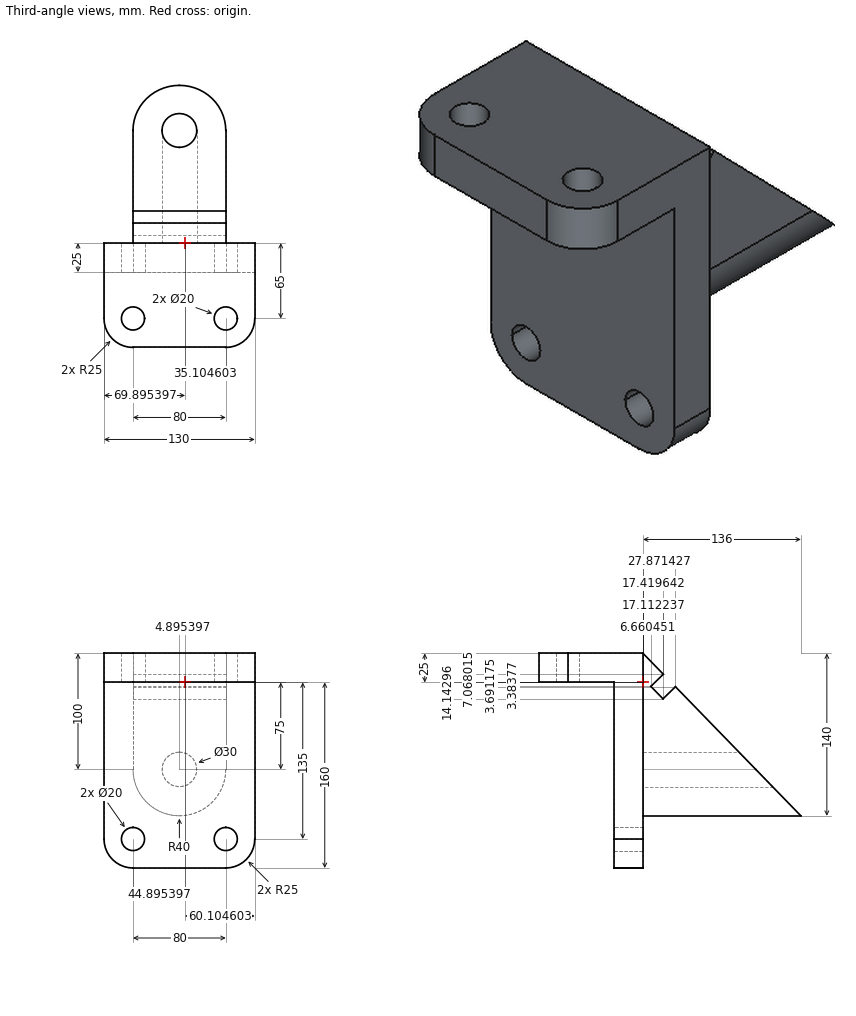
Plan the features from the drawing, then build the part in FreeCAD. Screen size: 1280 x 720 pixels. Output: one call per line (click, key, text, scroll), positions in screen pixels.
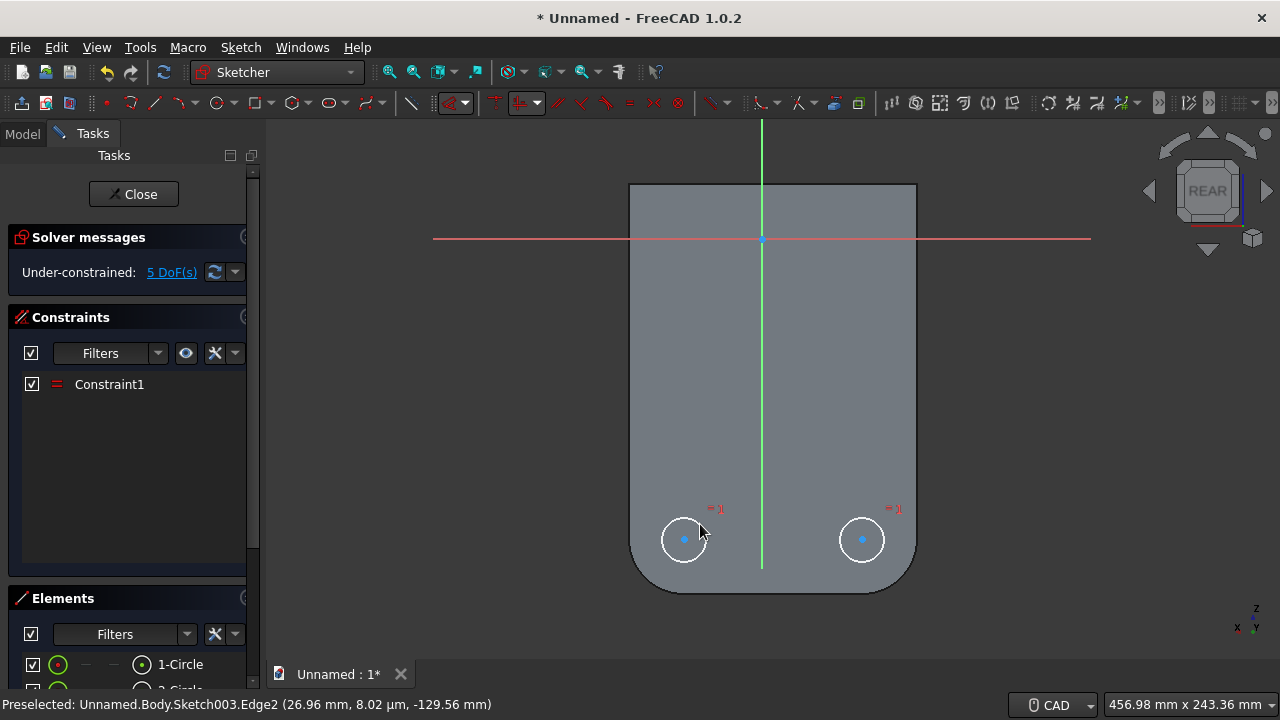
click(862, 540)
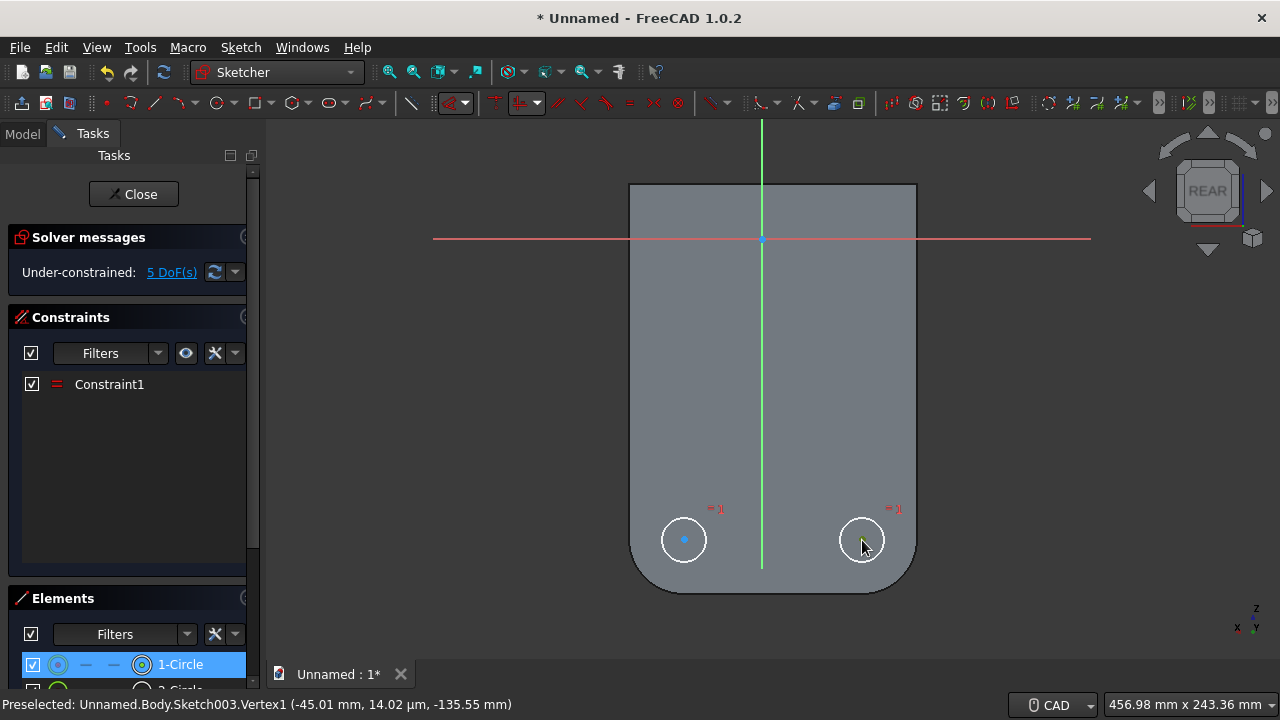
click(684, 540)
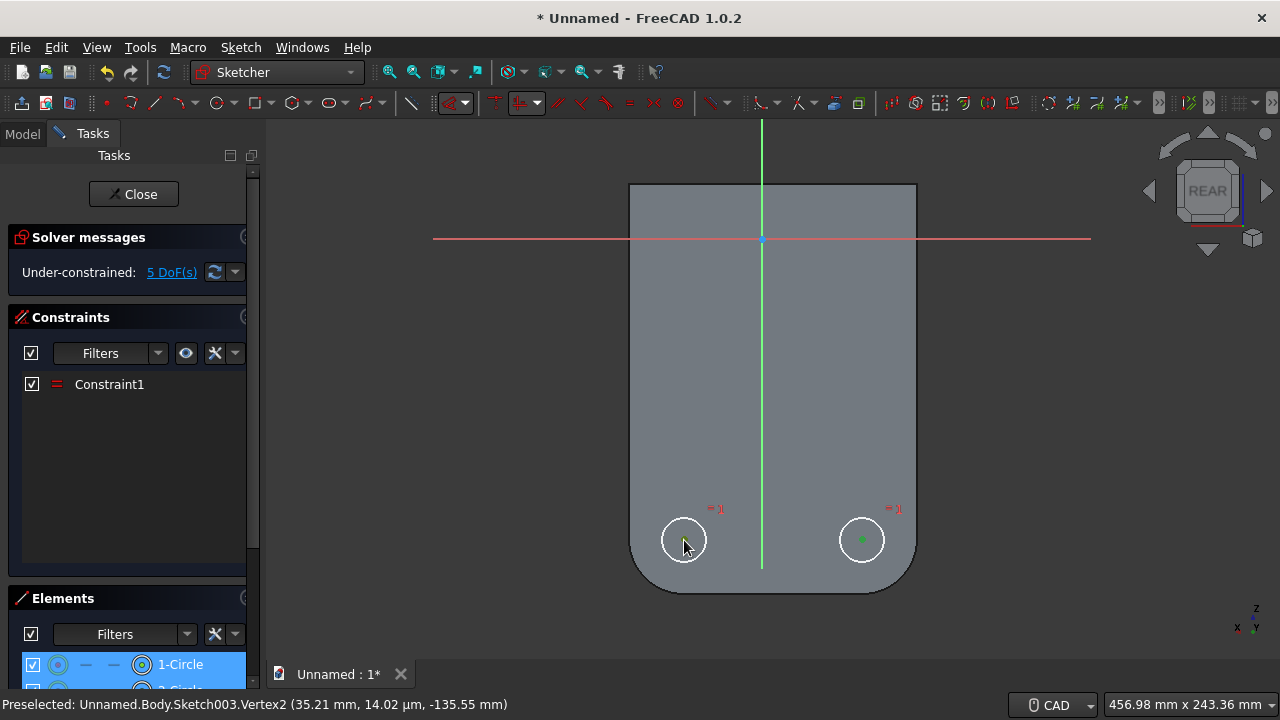
key(h)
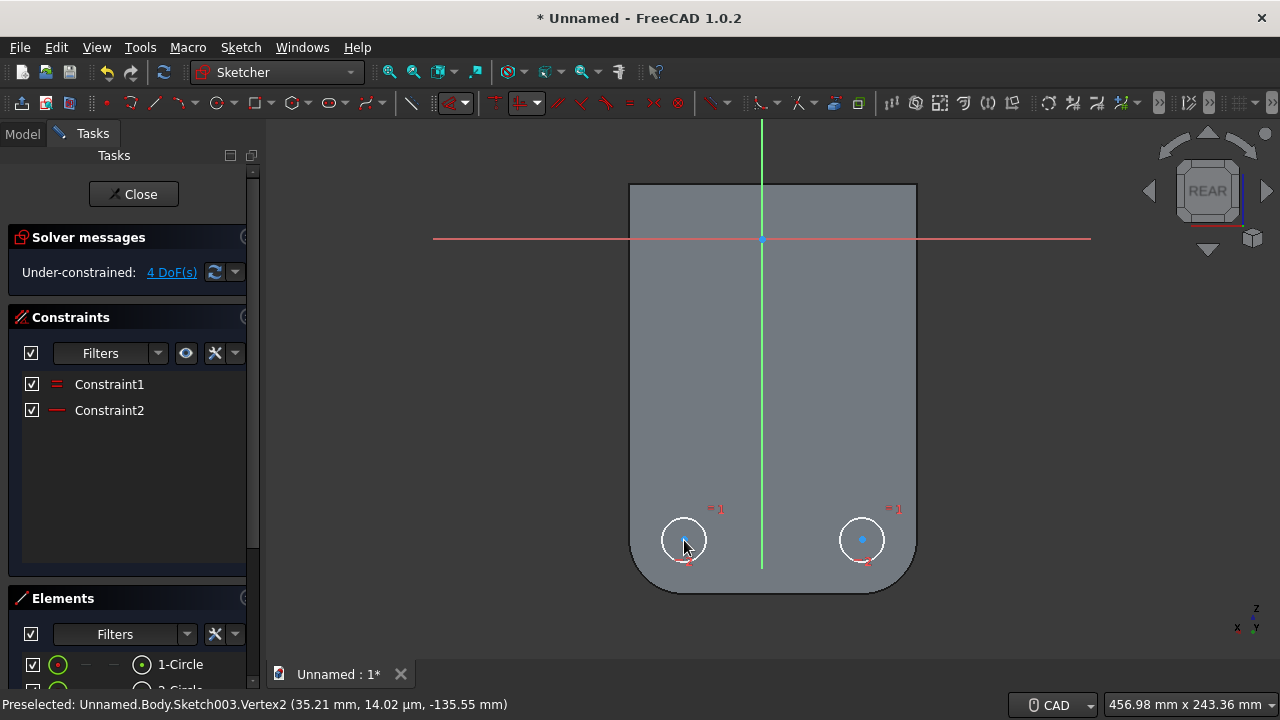
click(877, 524)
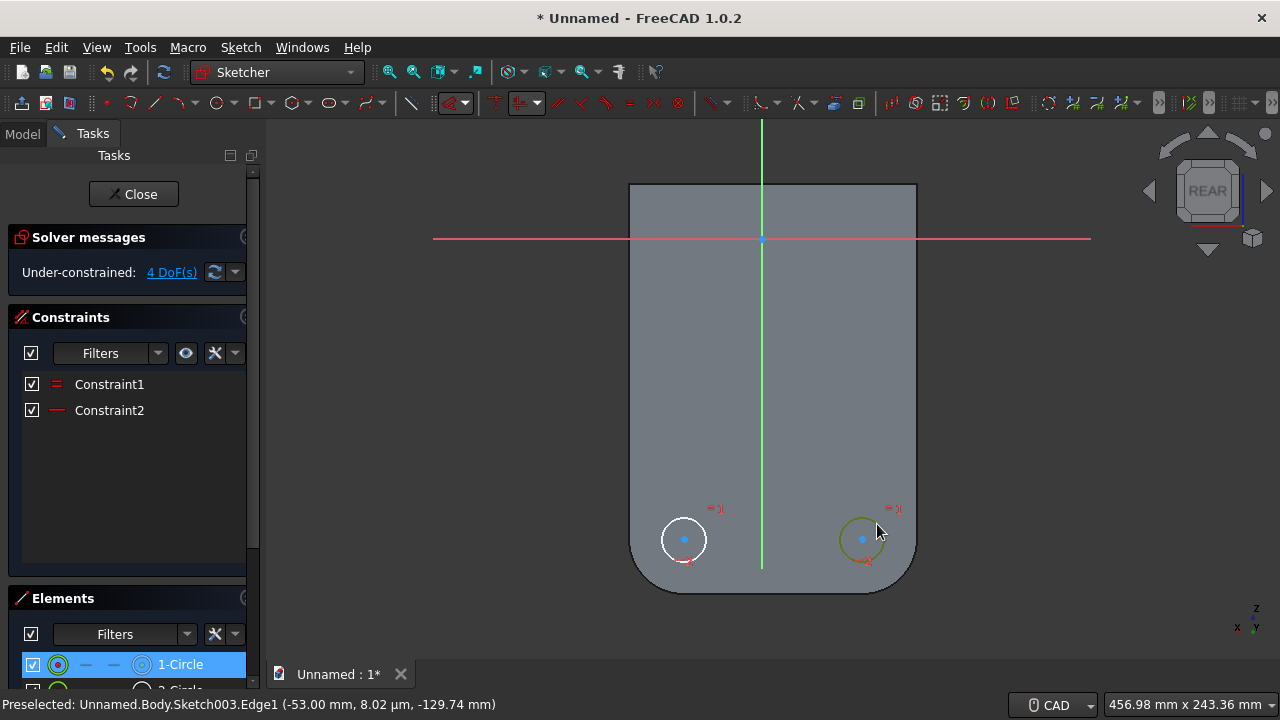
key(k)
key(o)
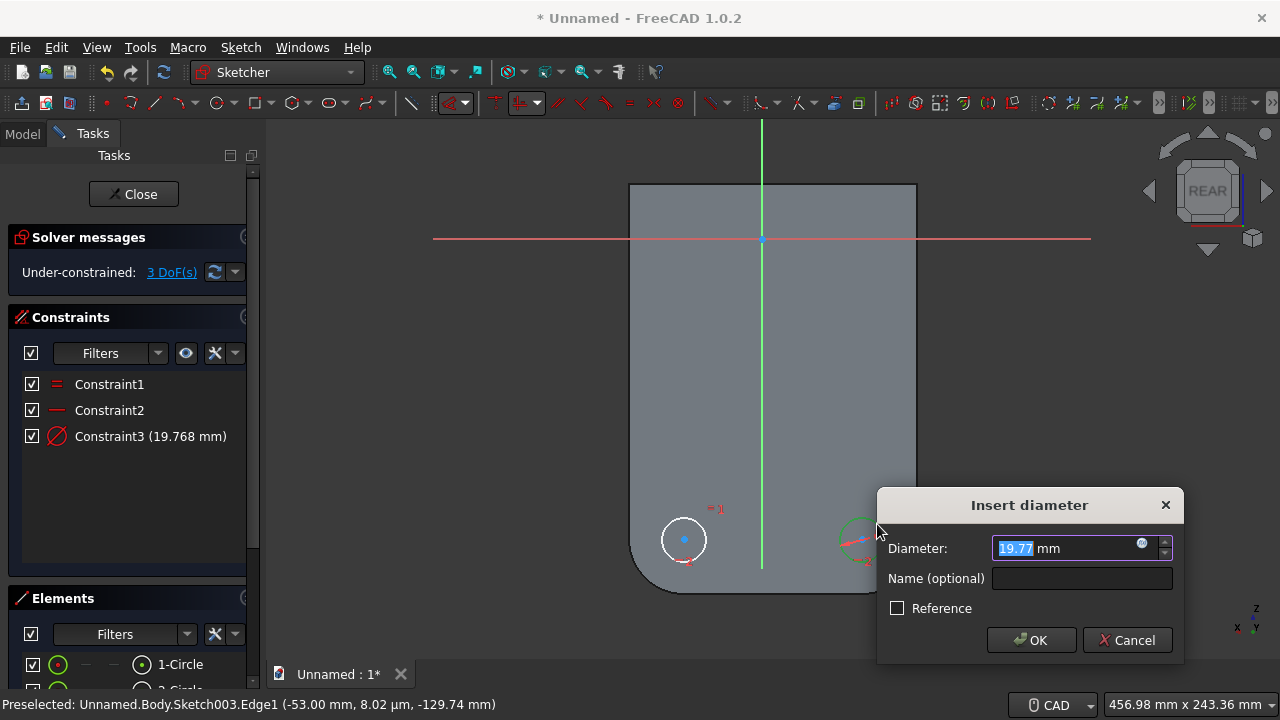
text(20)
key(Return)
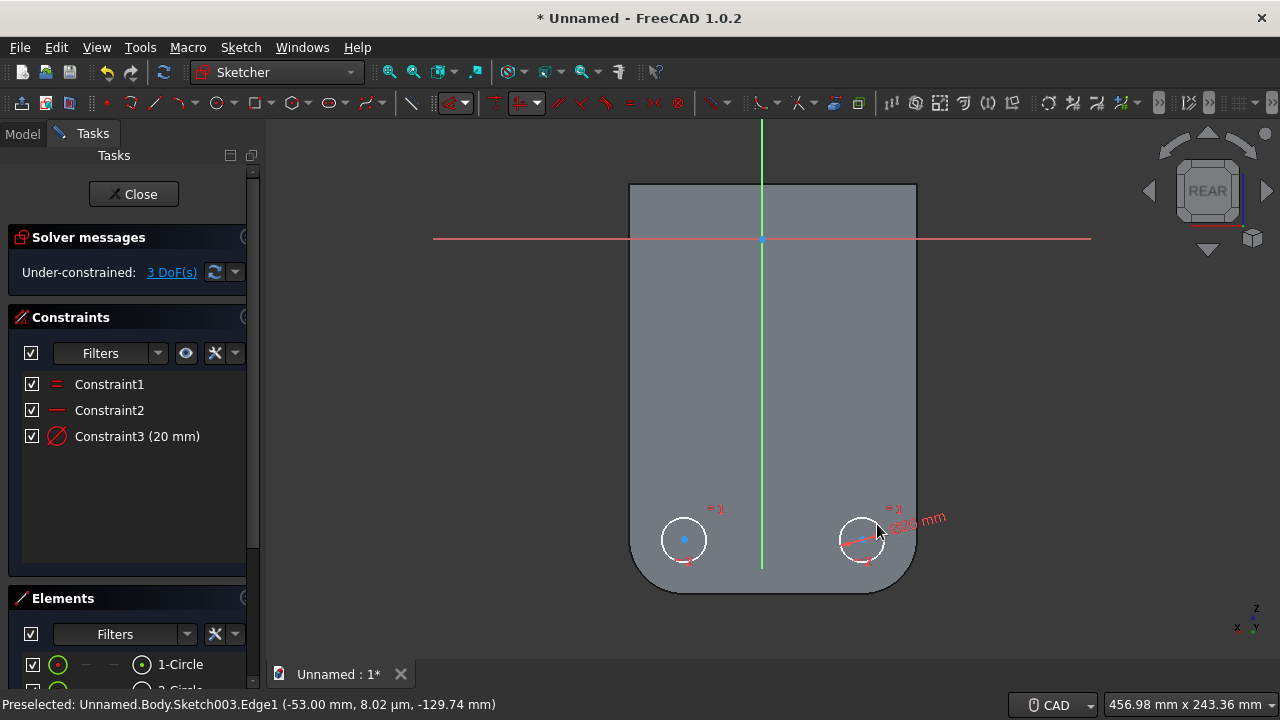
click(862, 540)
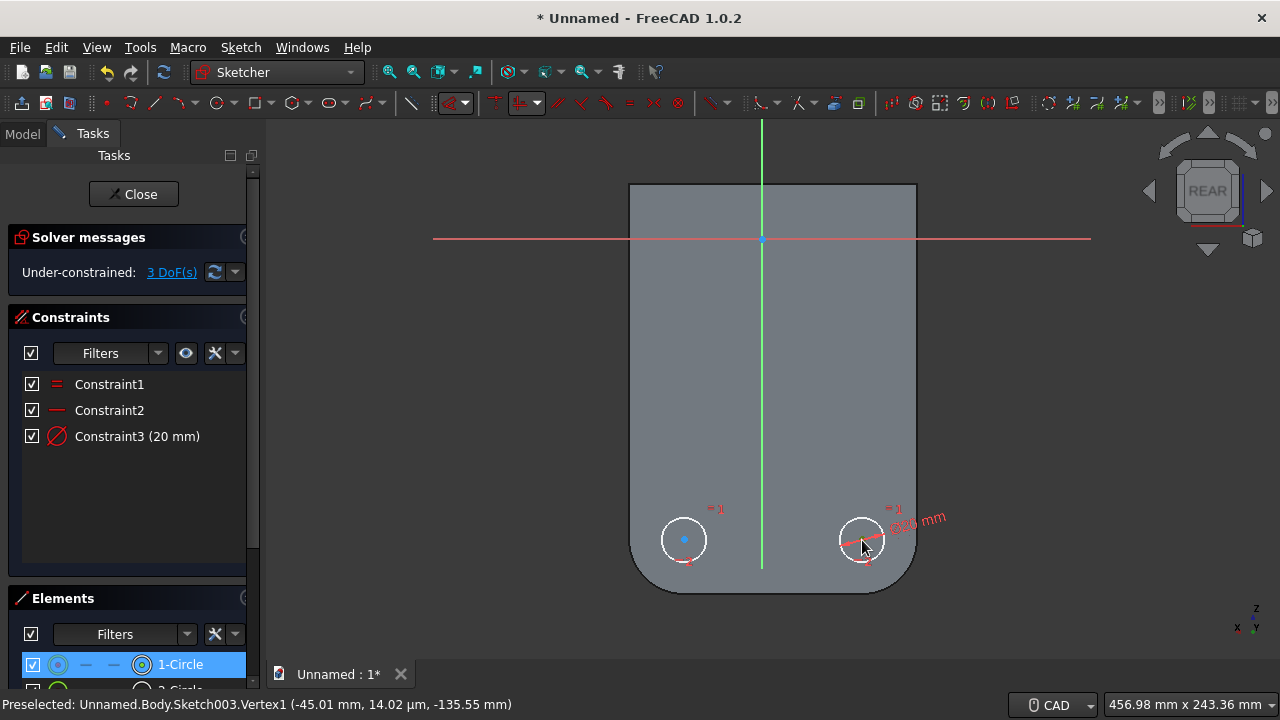
click(468, 104)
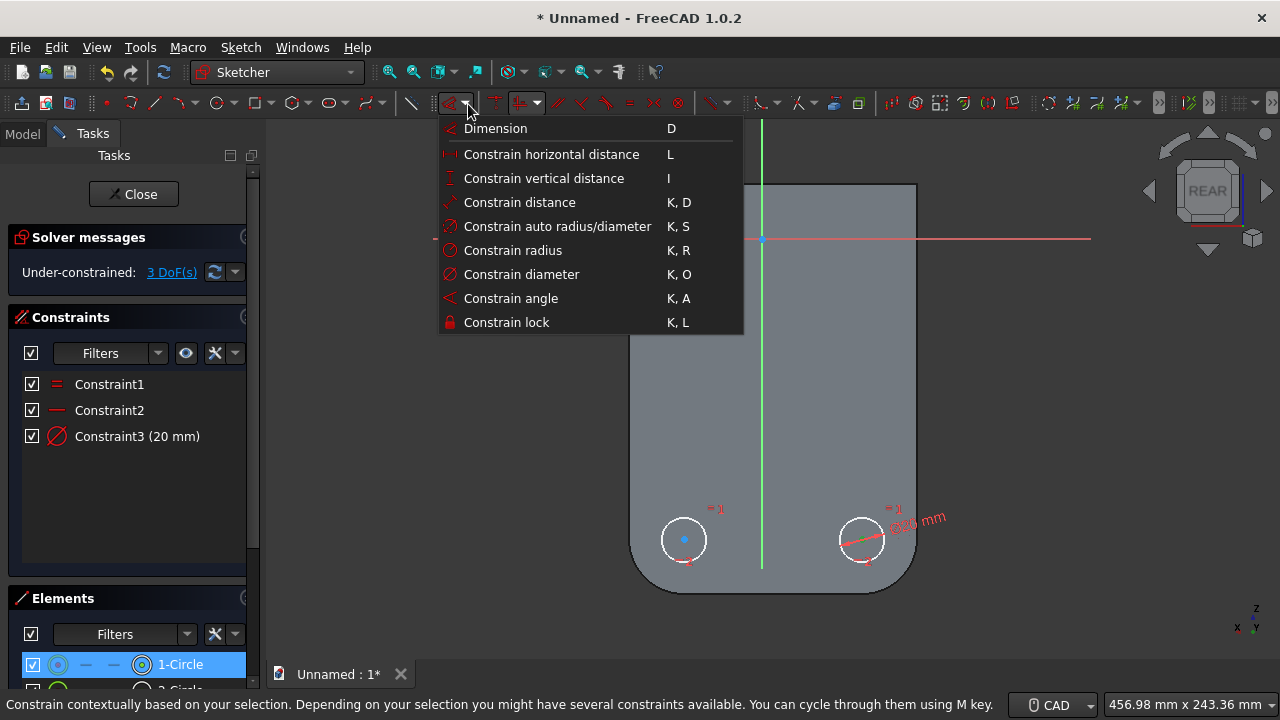
click(591, 178)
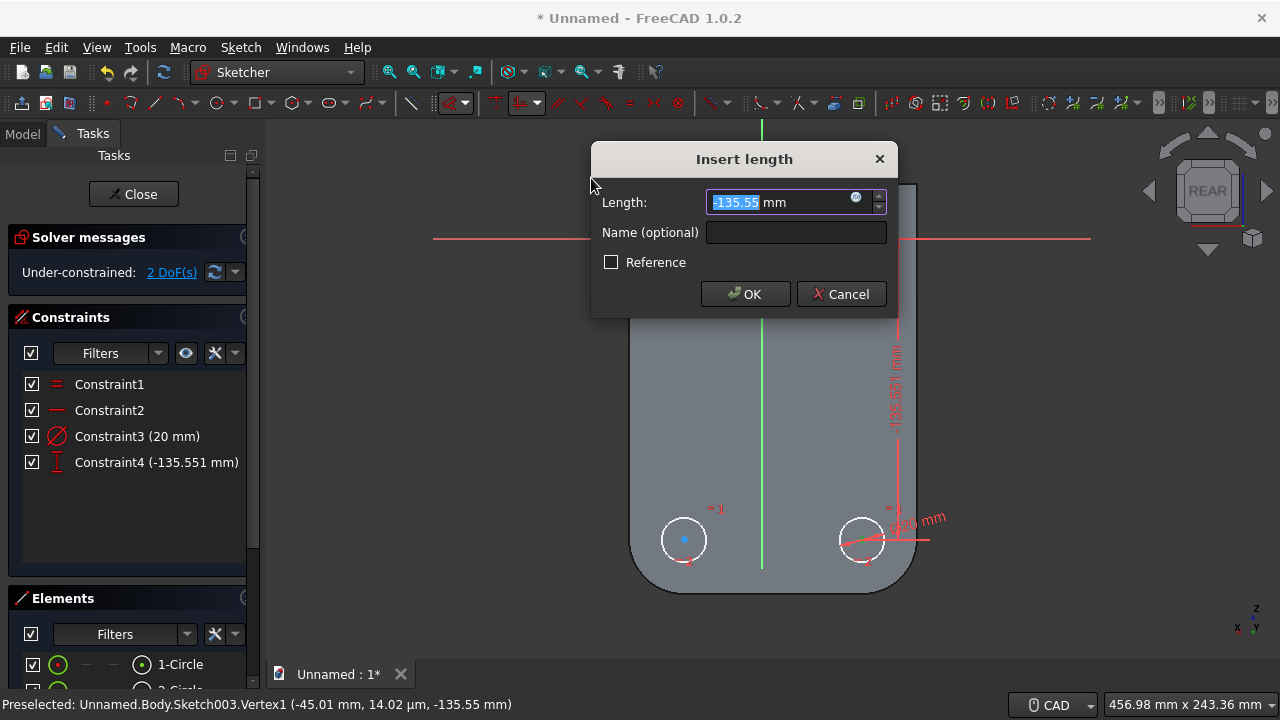
text(-135)
key(Return)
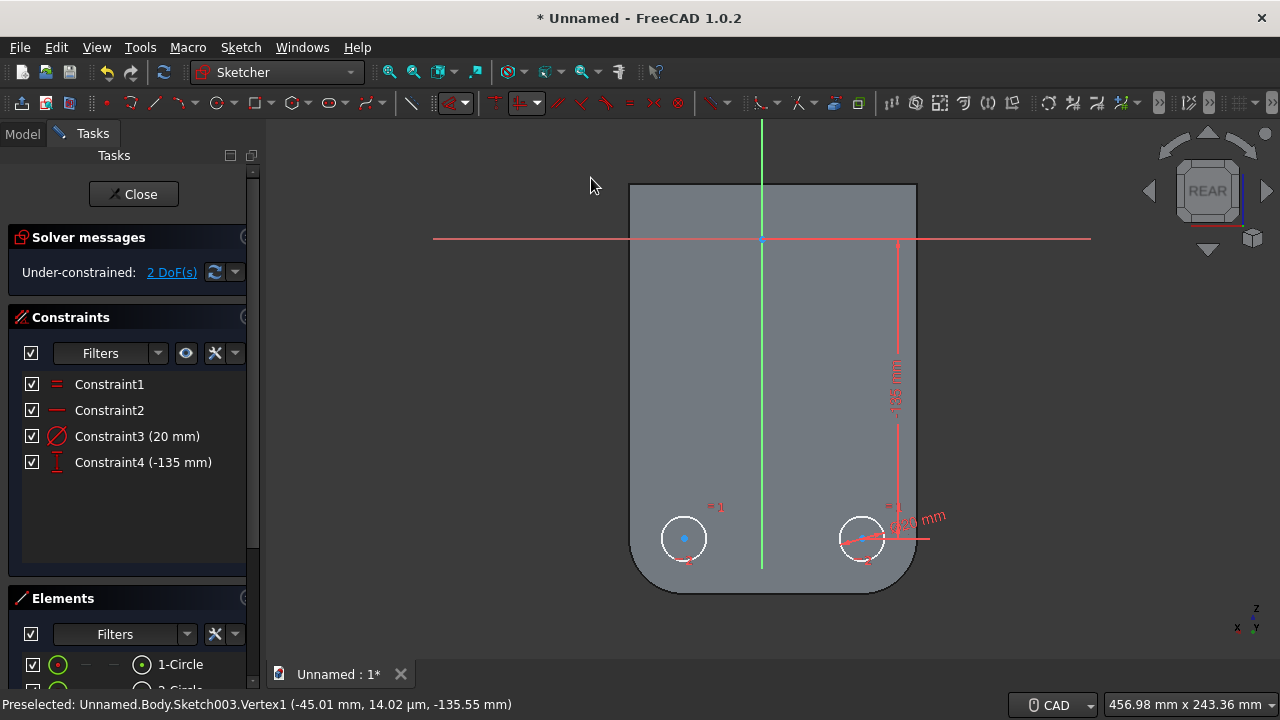
click(862, 539)